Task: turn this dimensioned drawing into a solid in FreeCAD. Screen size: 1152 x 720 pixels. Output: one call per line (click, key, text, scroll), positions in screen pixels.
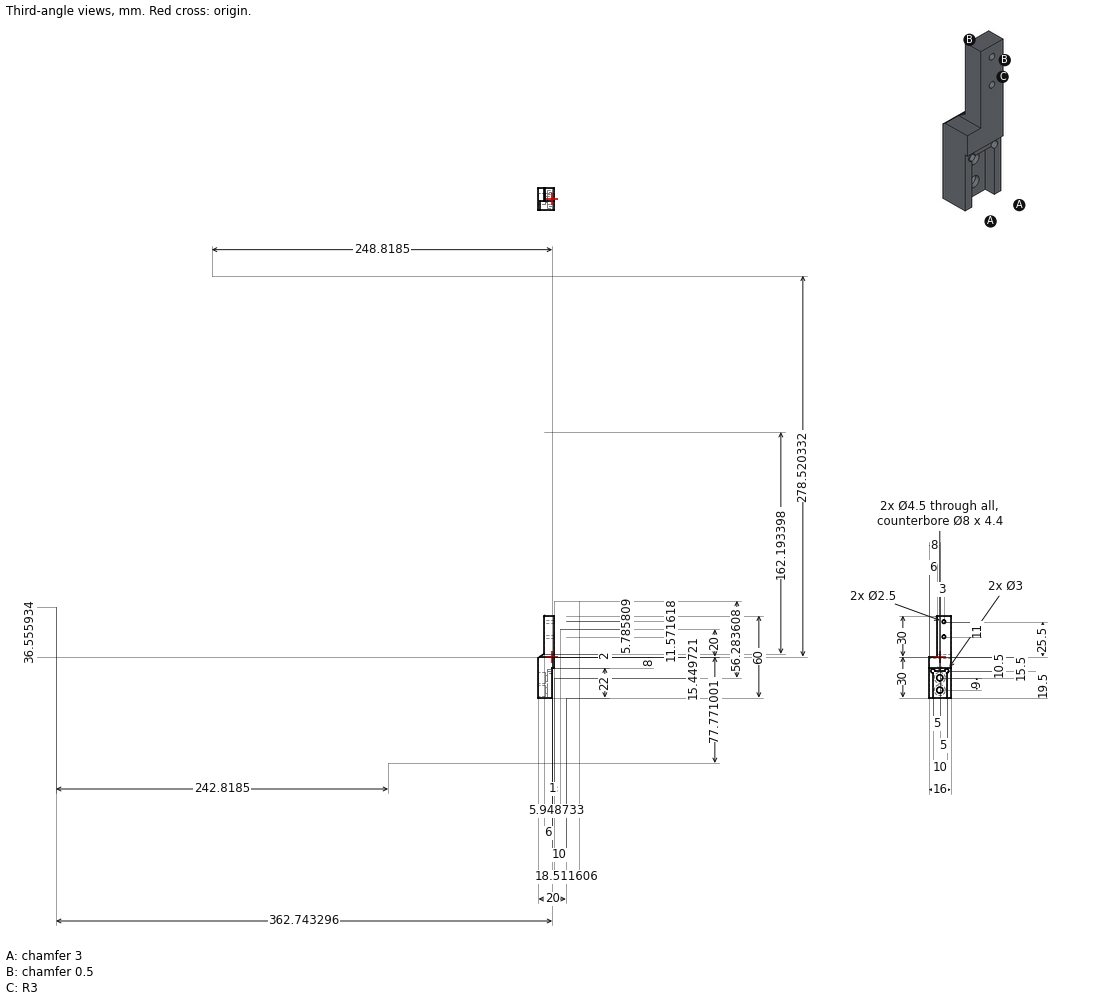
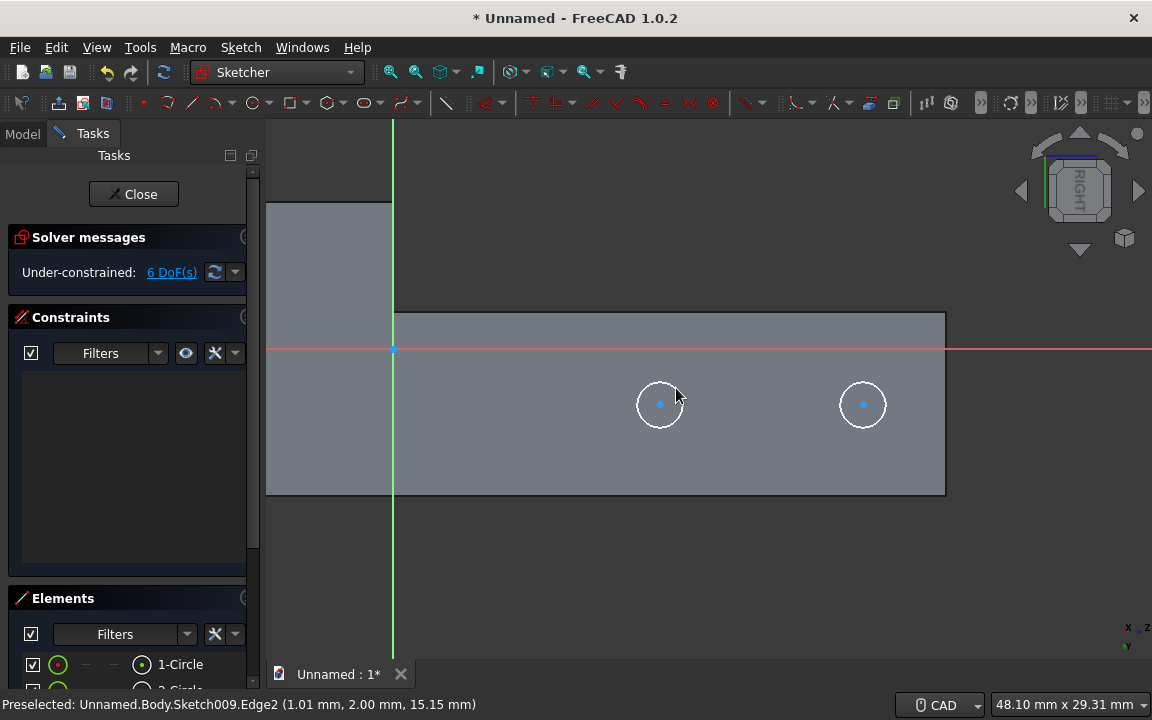
click(879, 389)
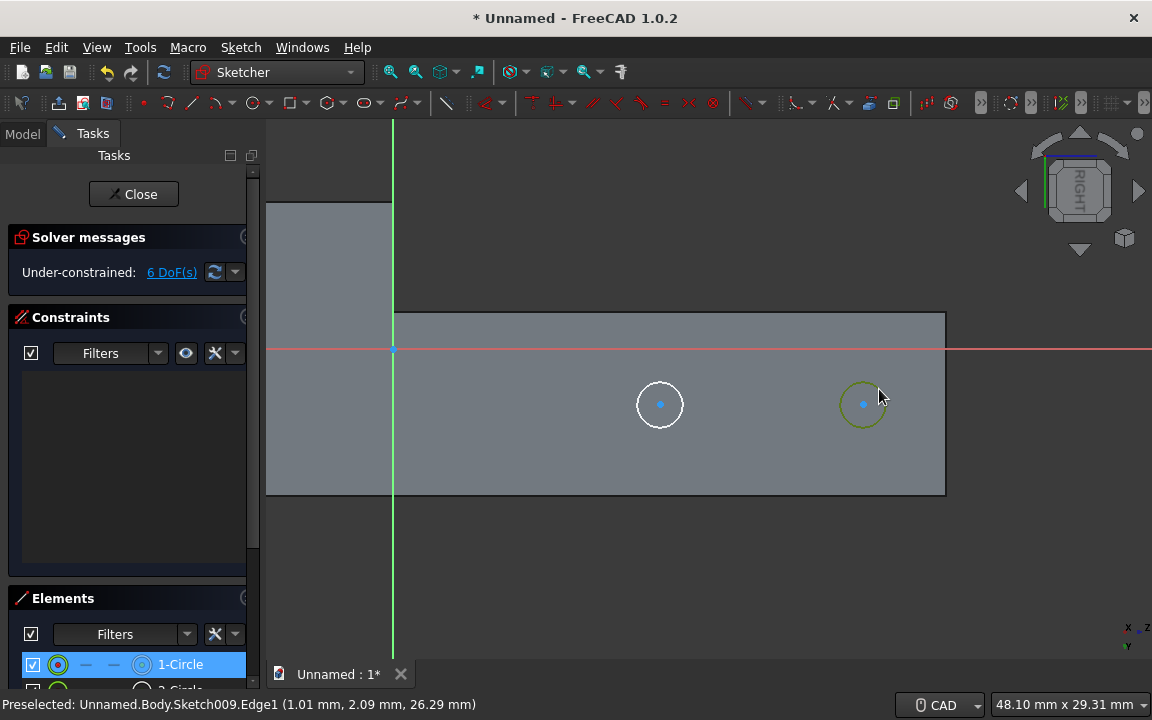
click(676, 389)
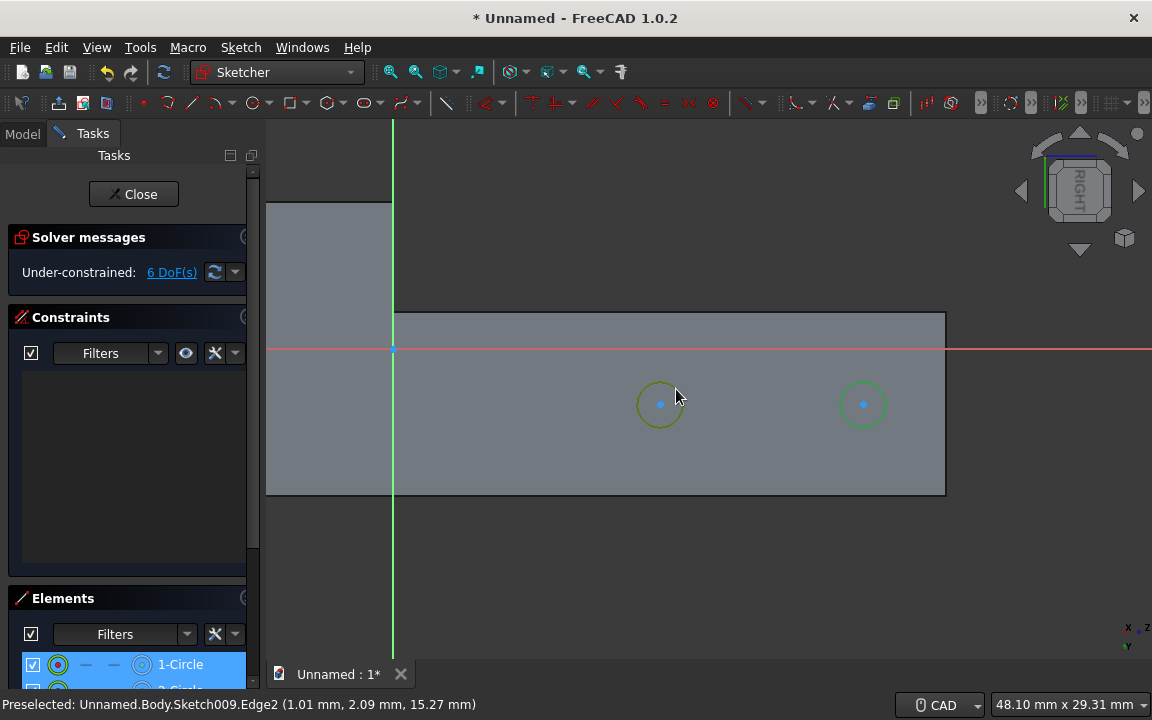
click(666, 104)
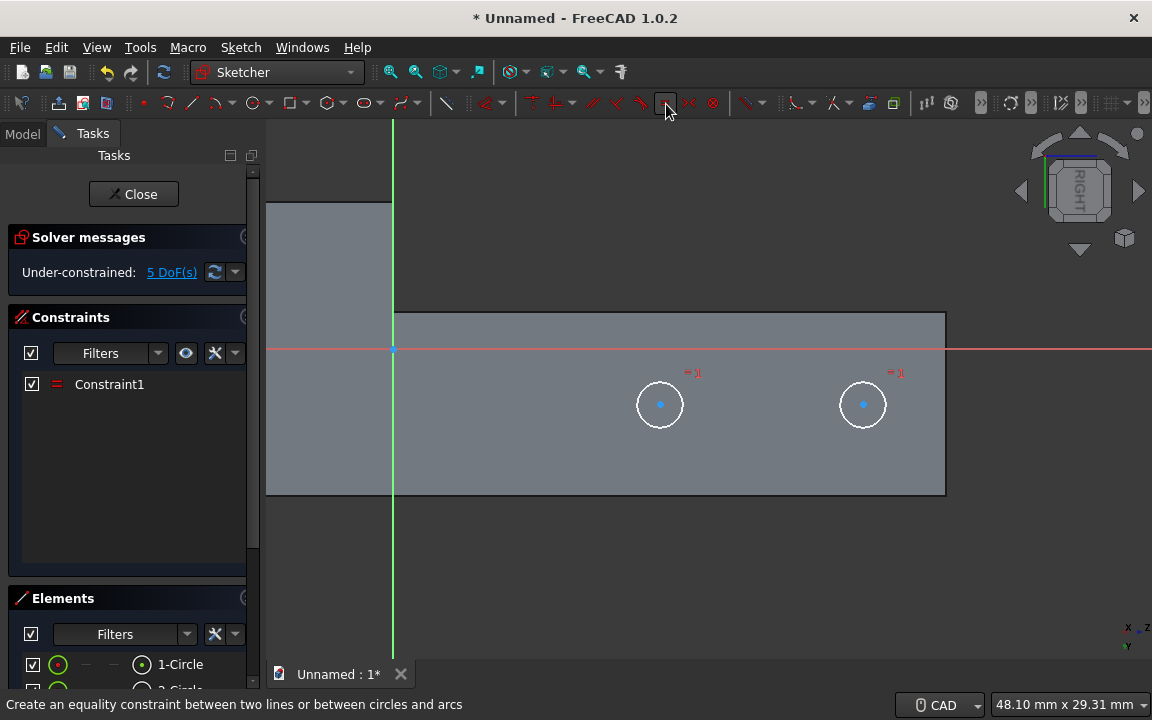
click(863, 405)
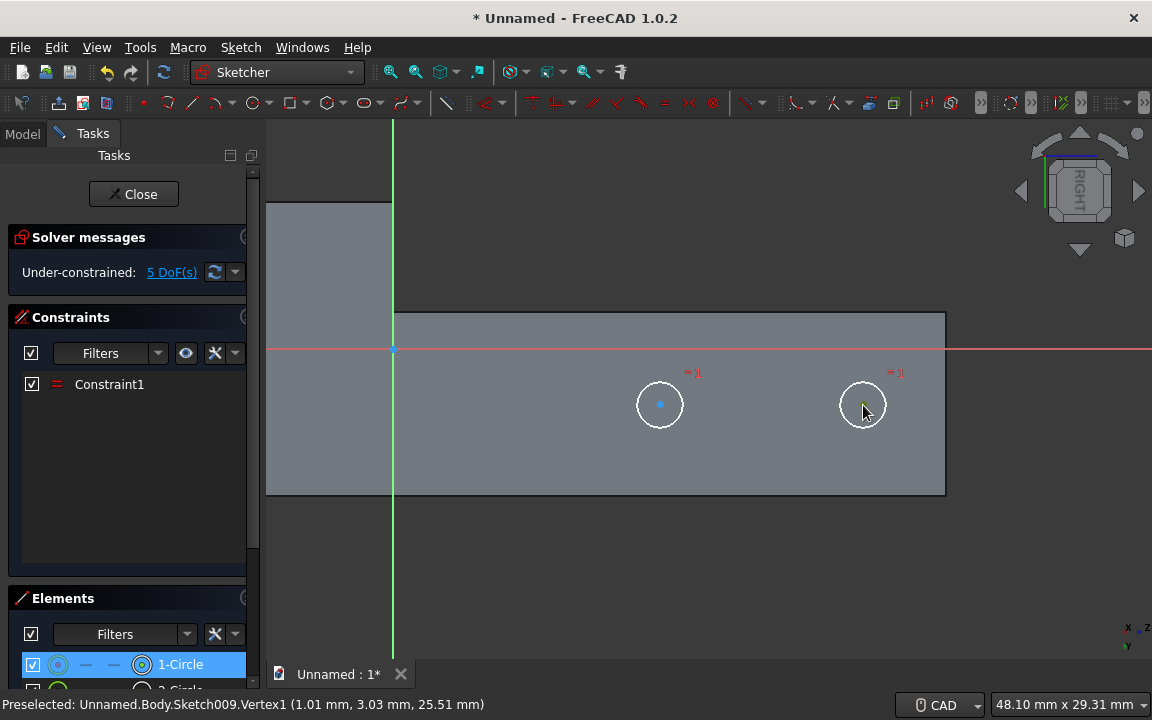
click(660, 405)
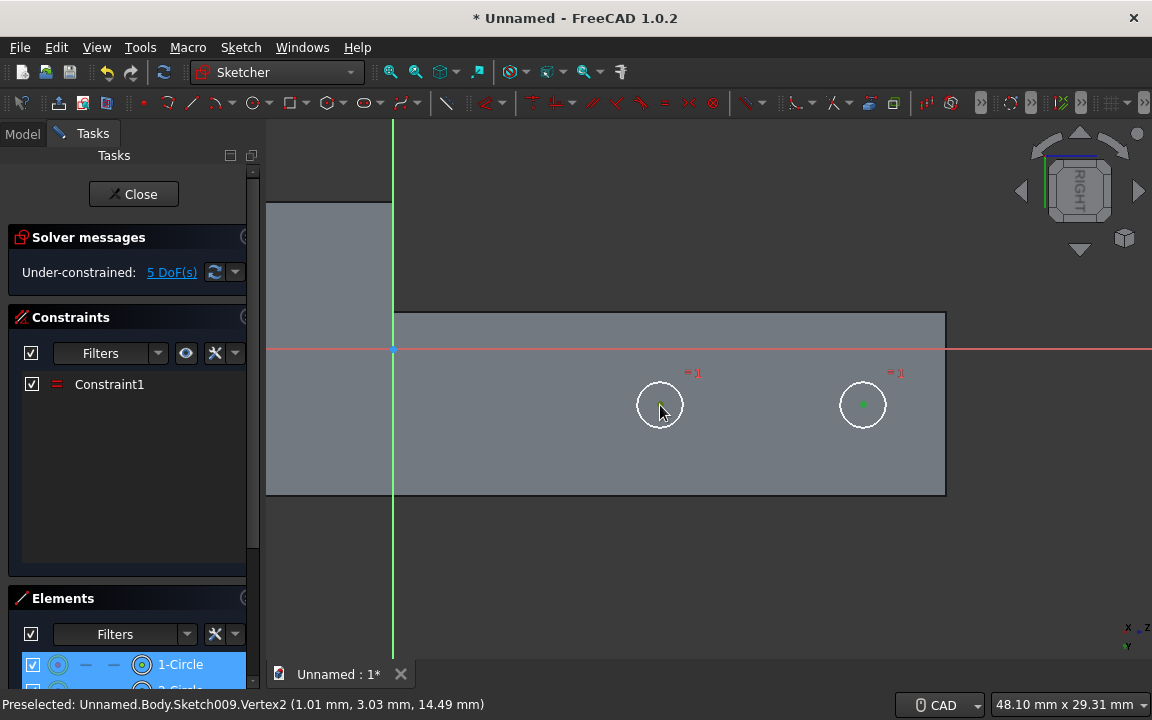
key(h)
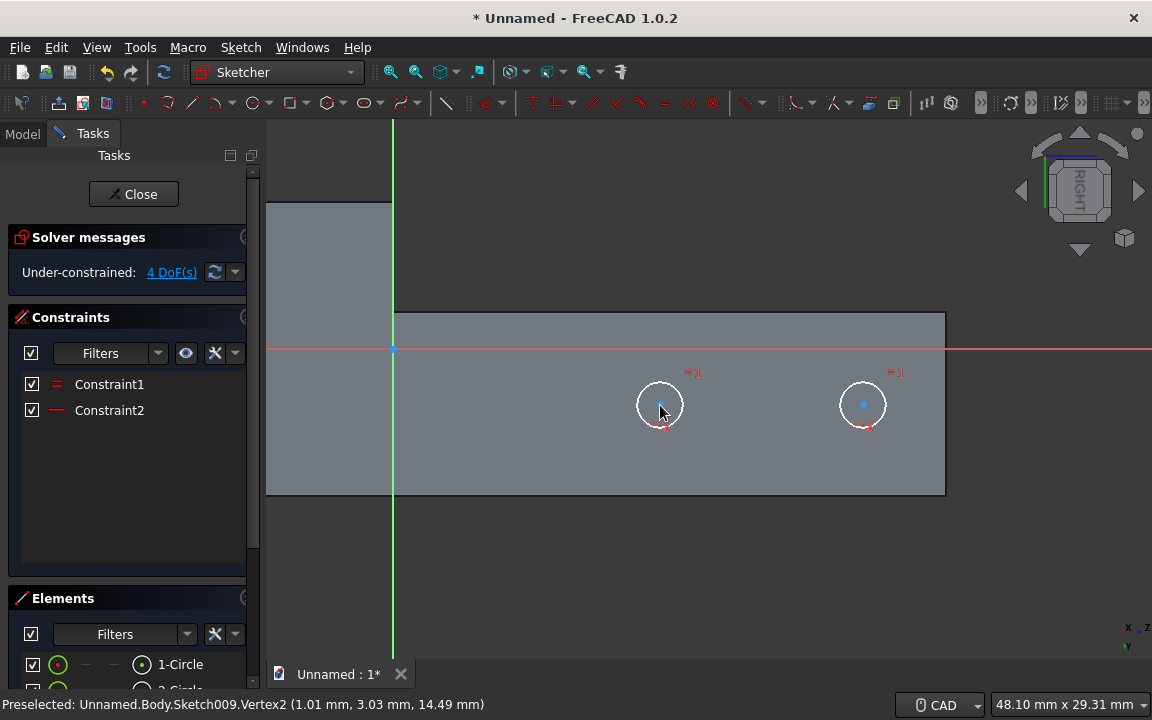
click(486, 104)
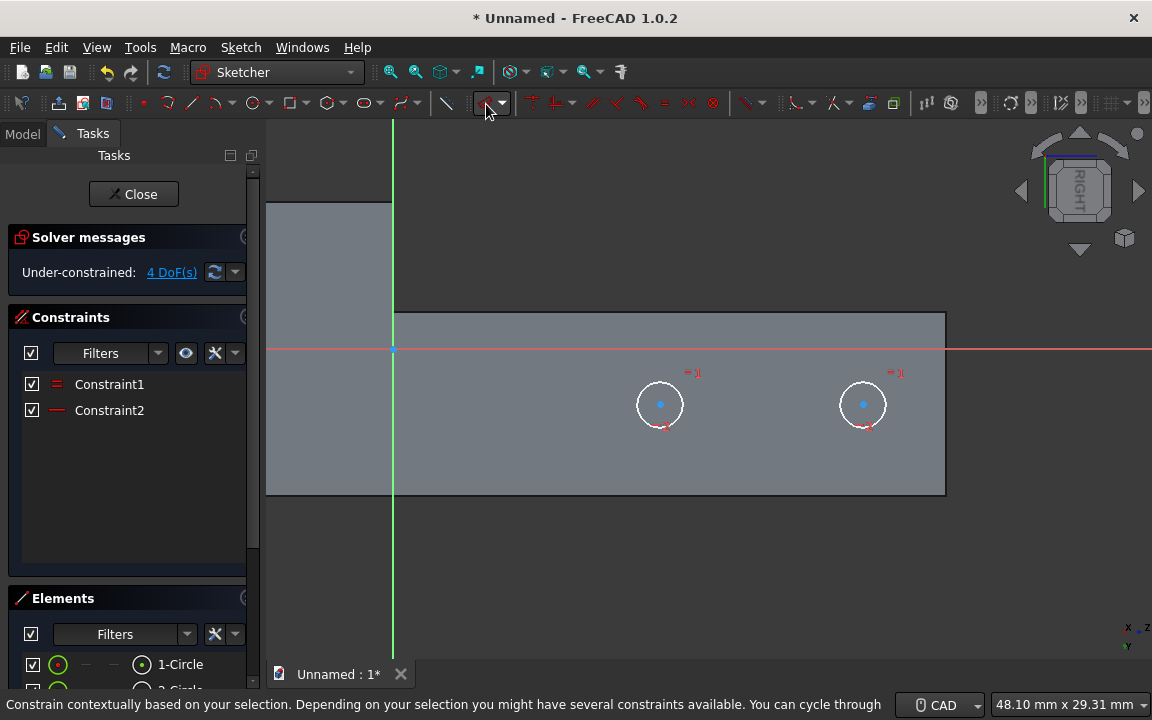
click(879, 389)
click(902, 366)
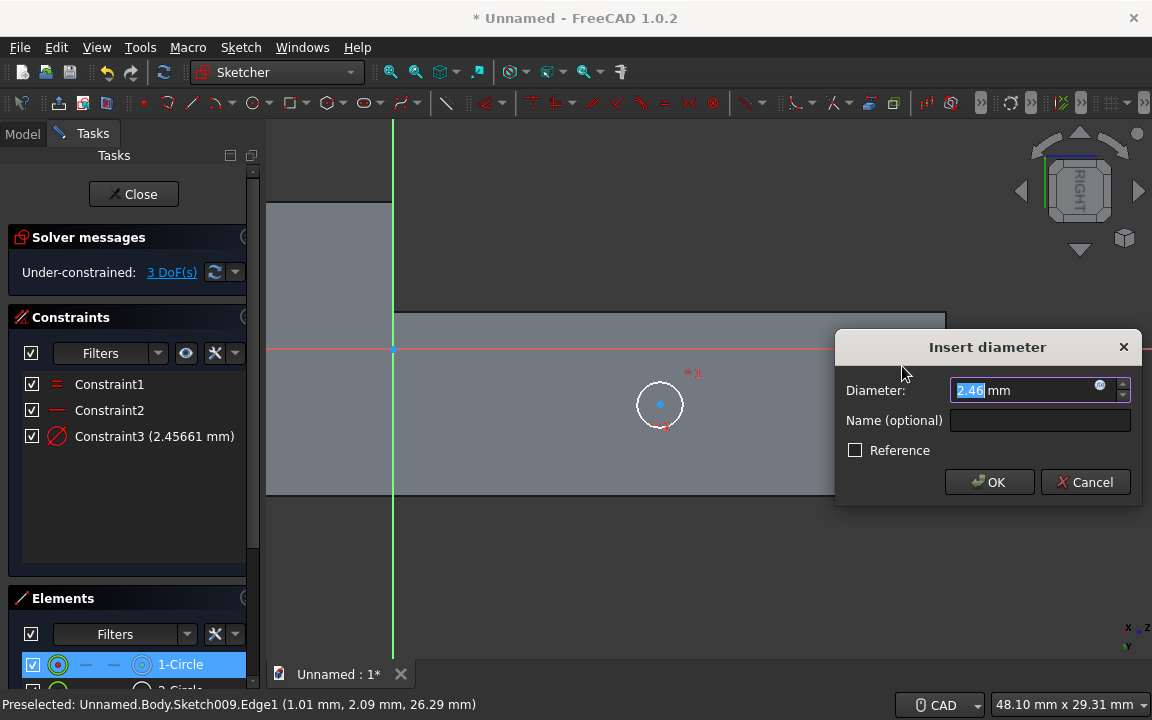
text(2.5)
key(Return)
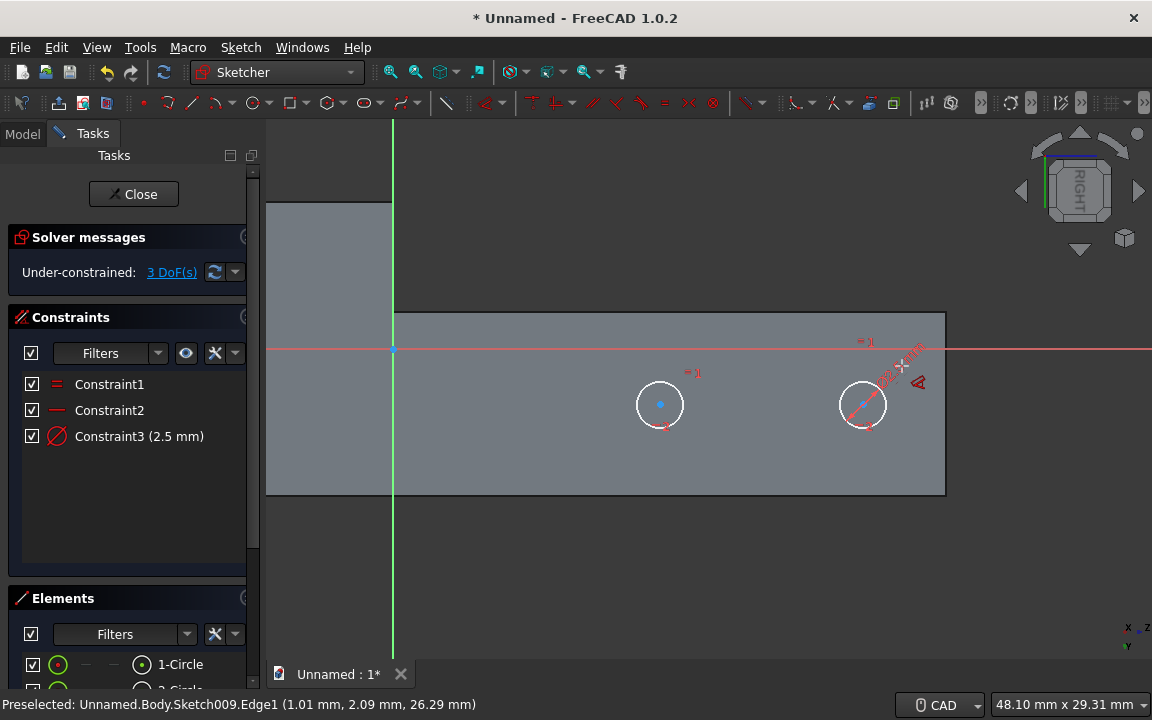
click(863, 405)
click(359, 377)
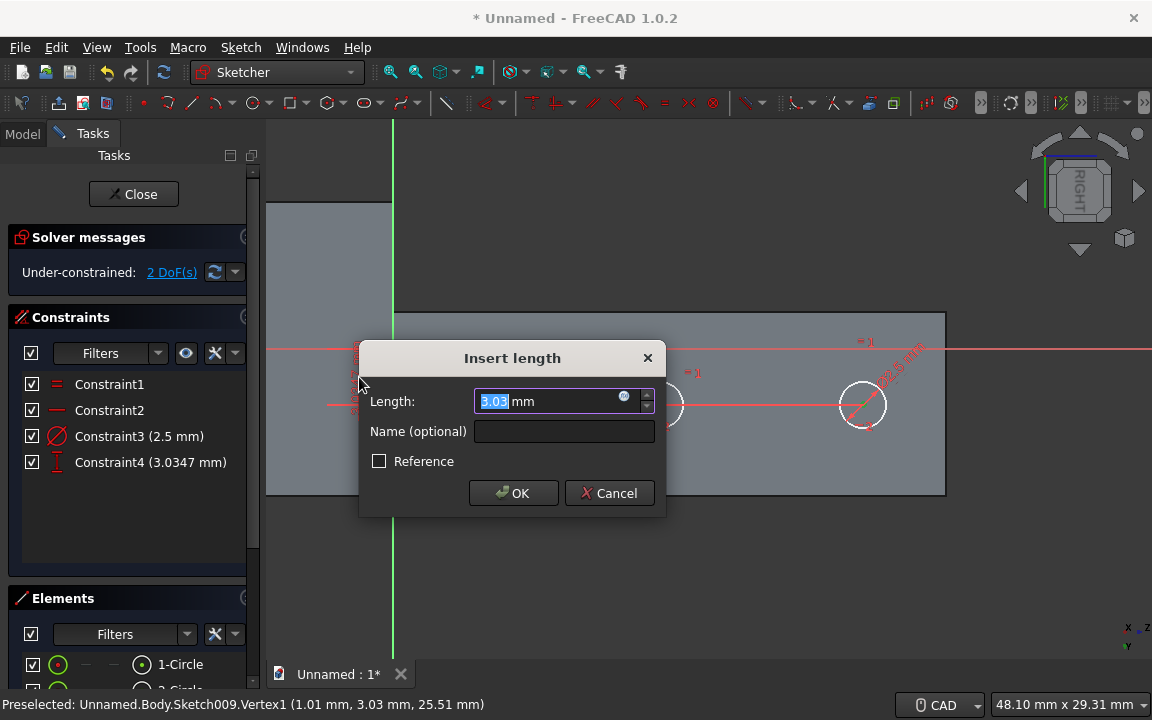
text(3)
key(Return)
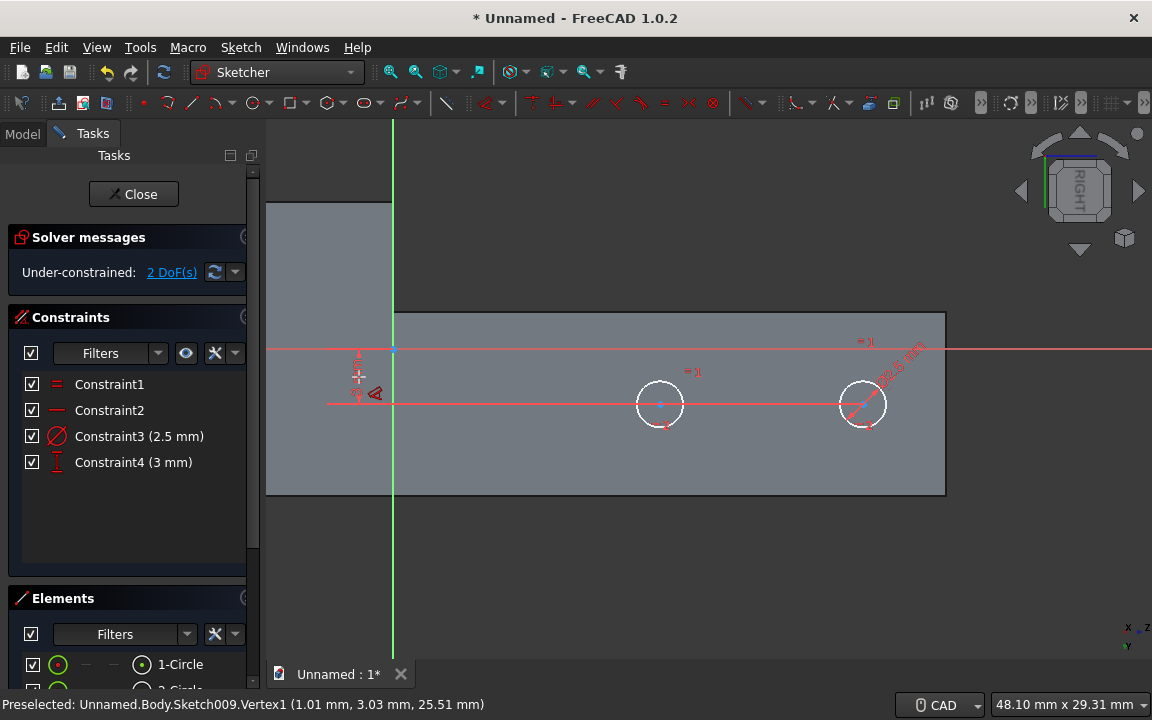
click(863, 404)